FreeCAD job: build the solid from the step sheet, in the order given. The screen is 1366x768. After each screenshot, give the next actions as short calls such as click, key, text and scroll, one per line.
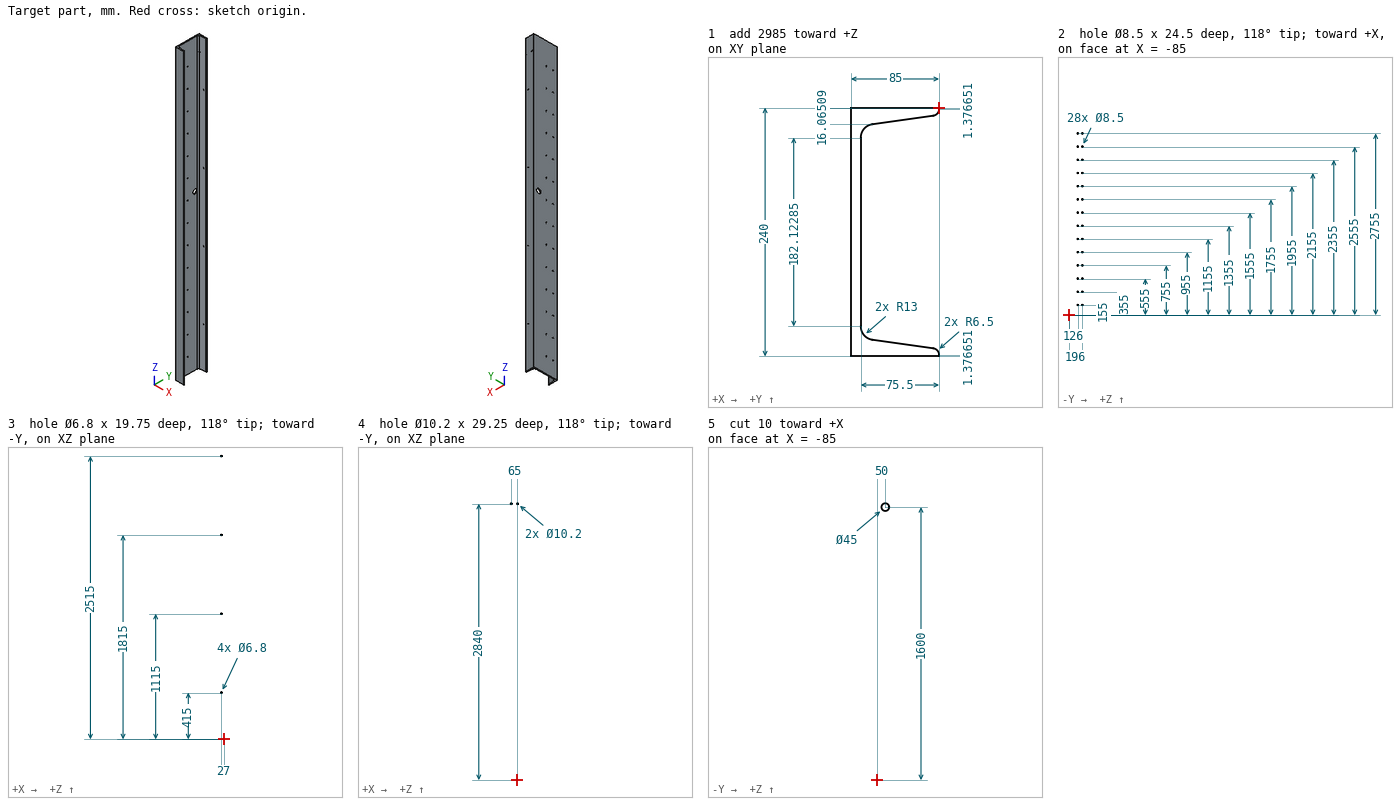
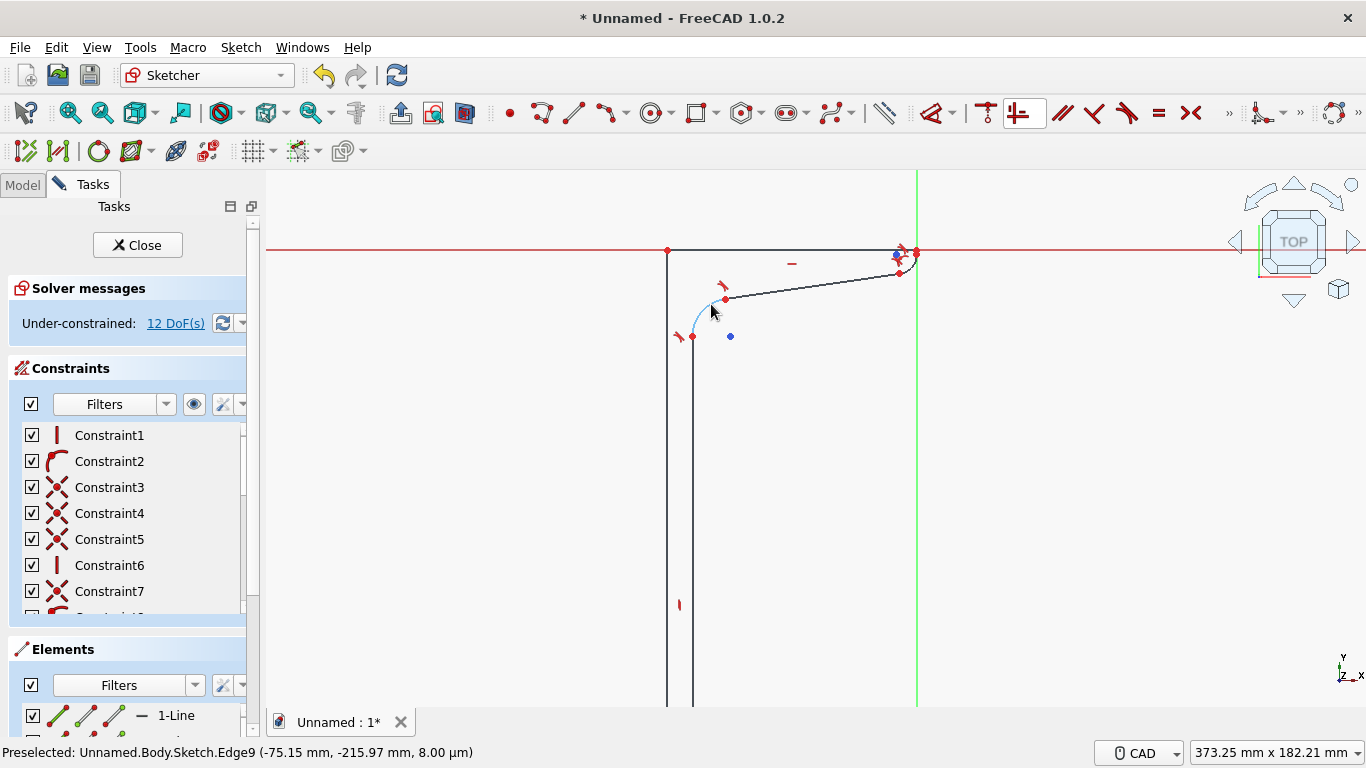
click(710, 305)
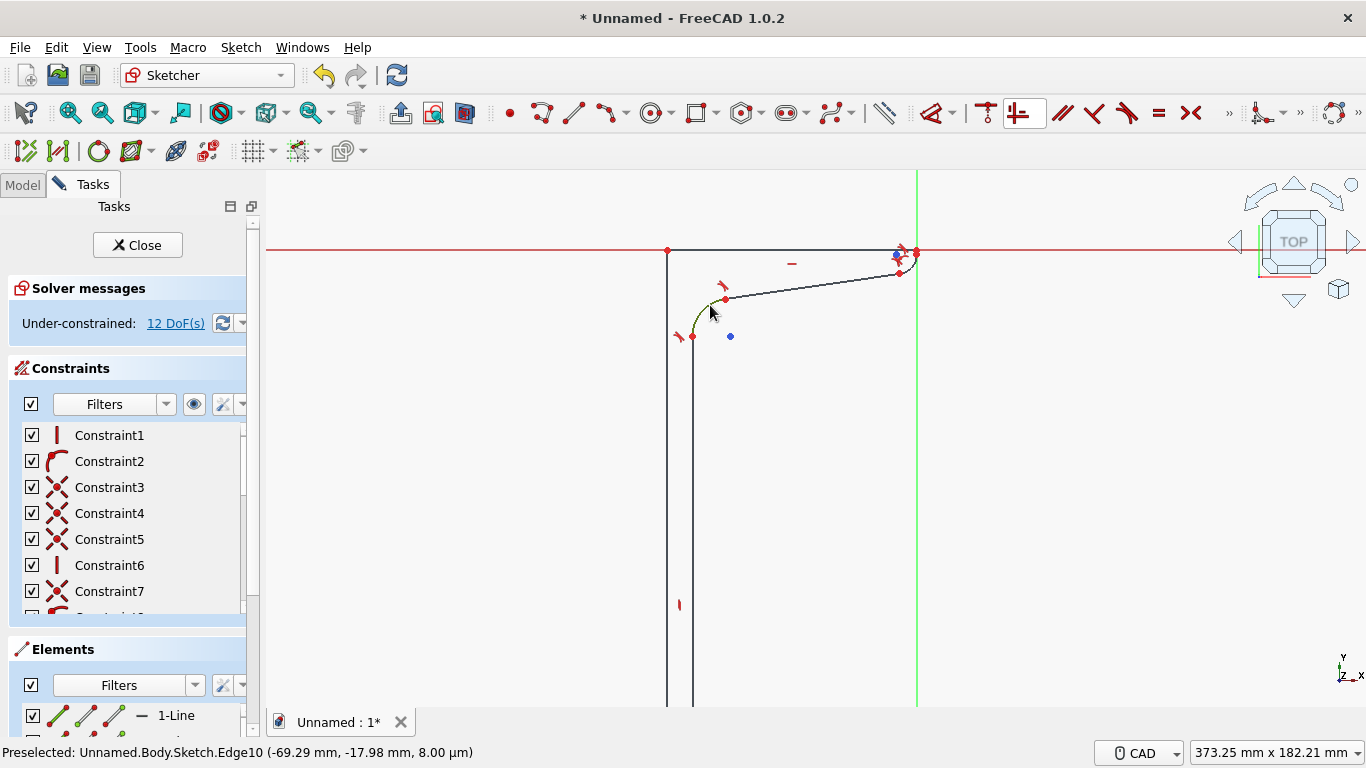
click(1160, 114)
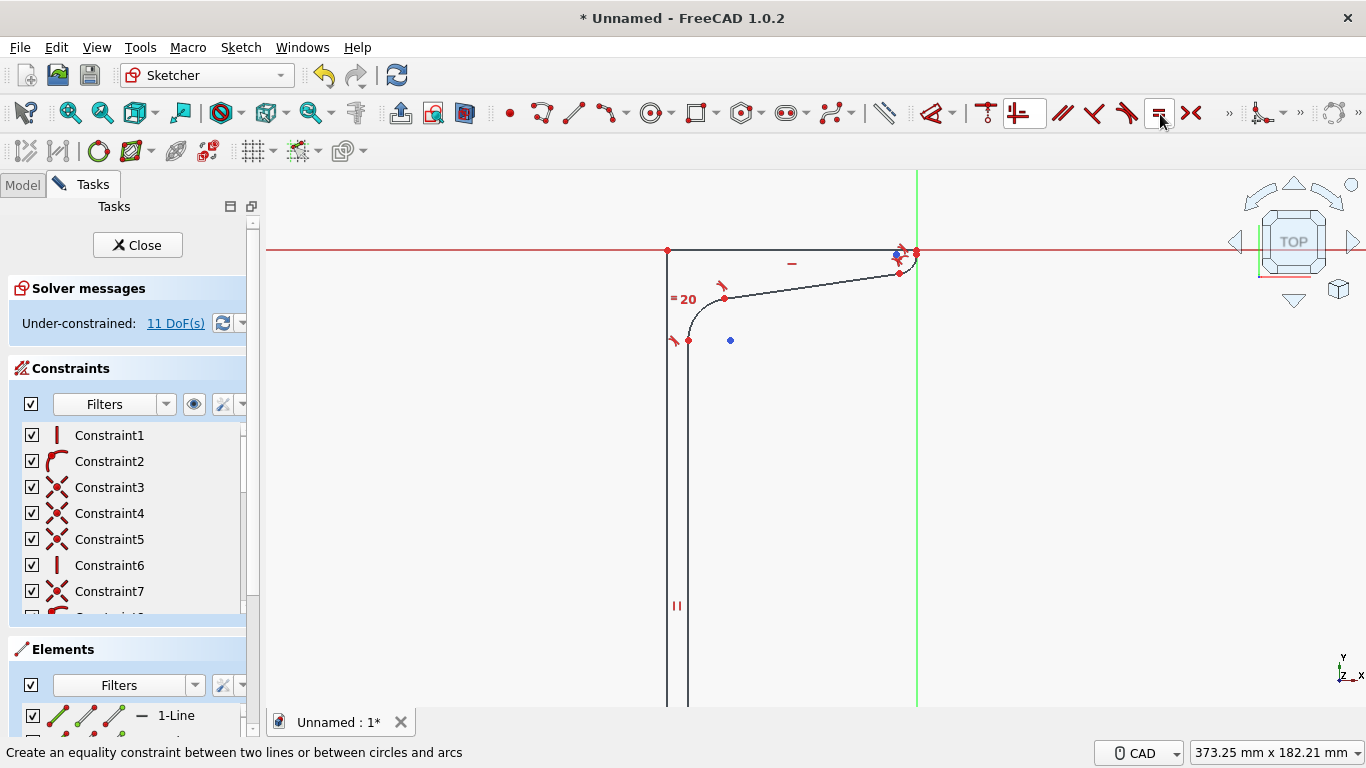
scroll(915, 262, up, 3)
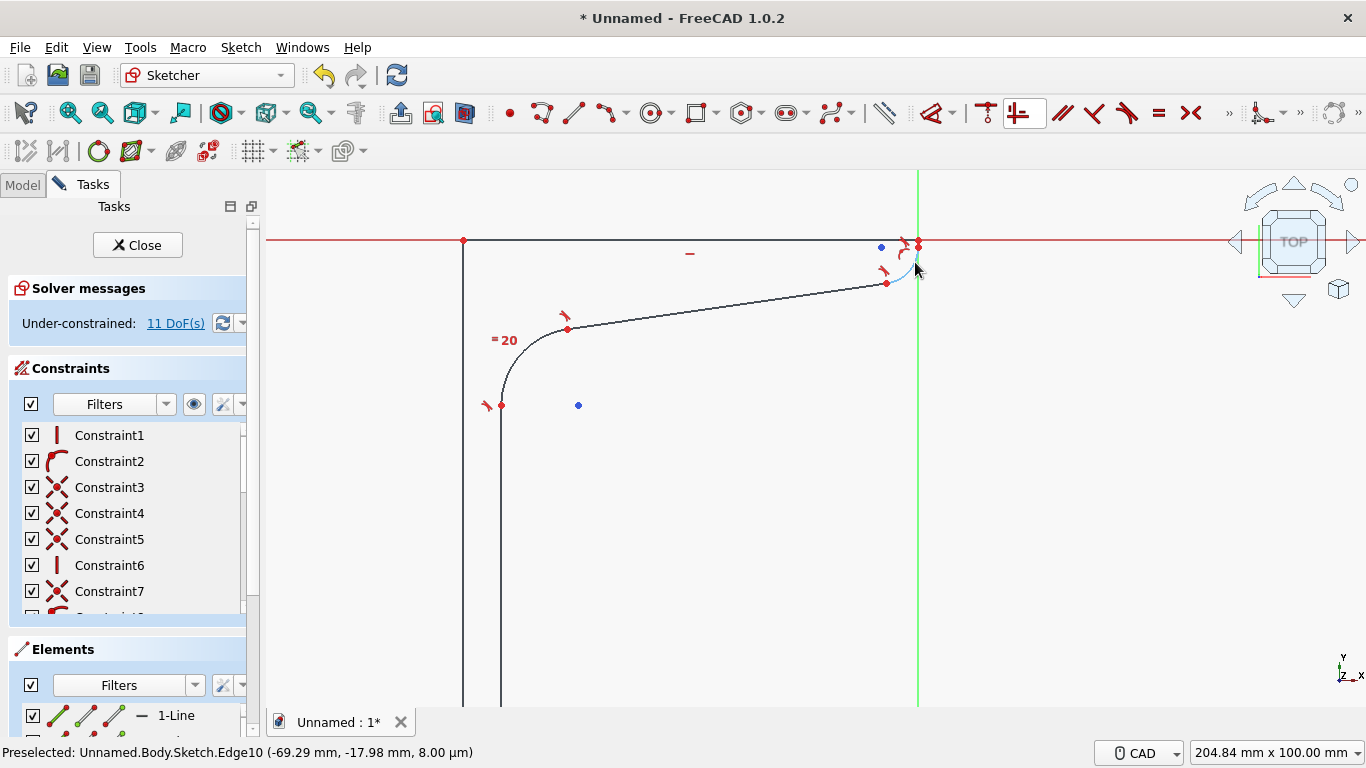
click(915, 263)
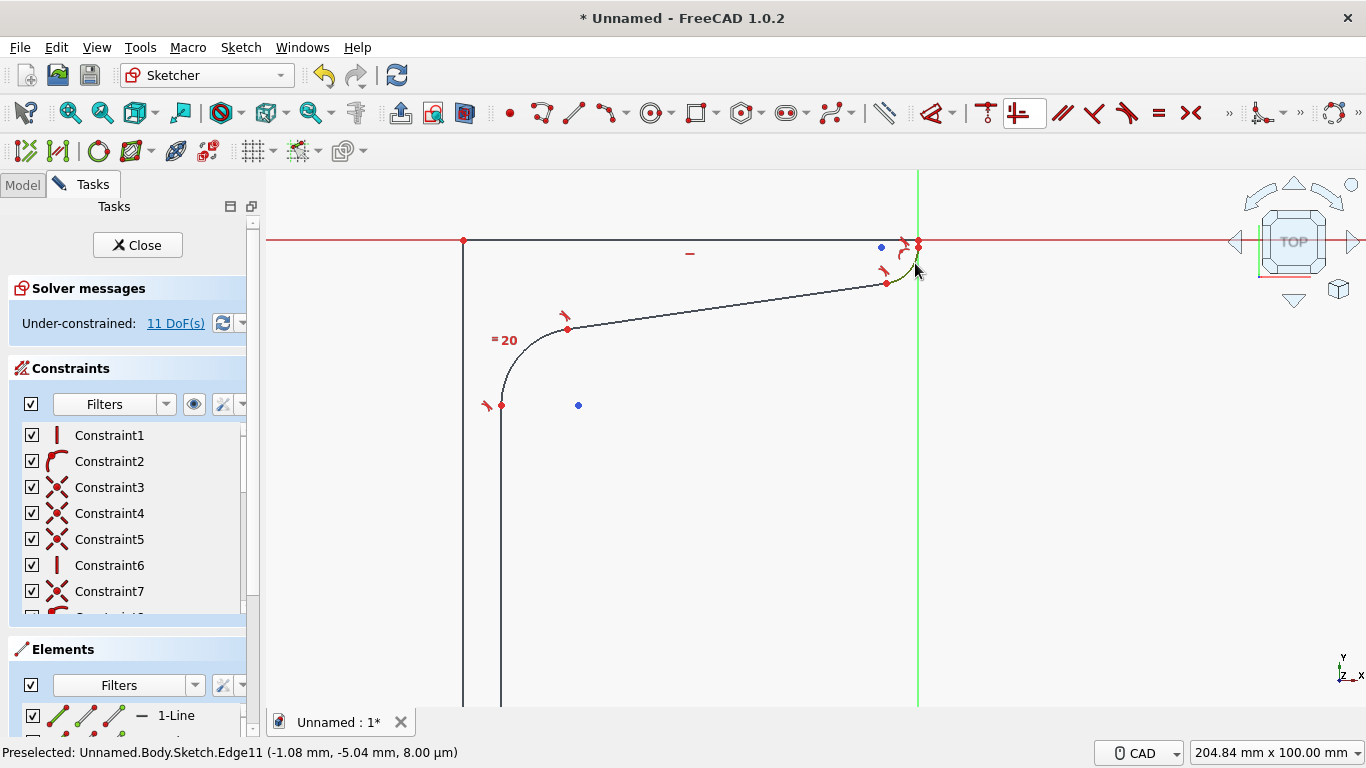
scroll(766, 293, down, 7)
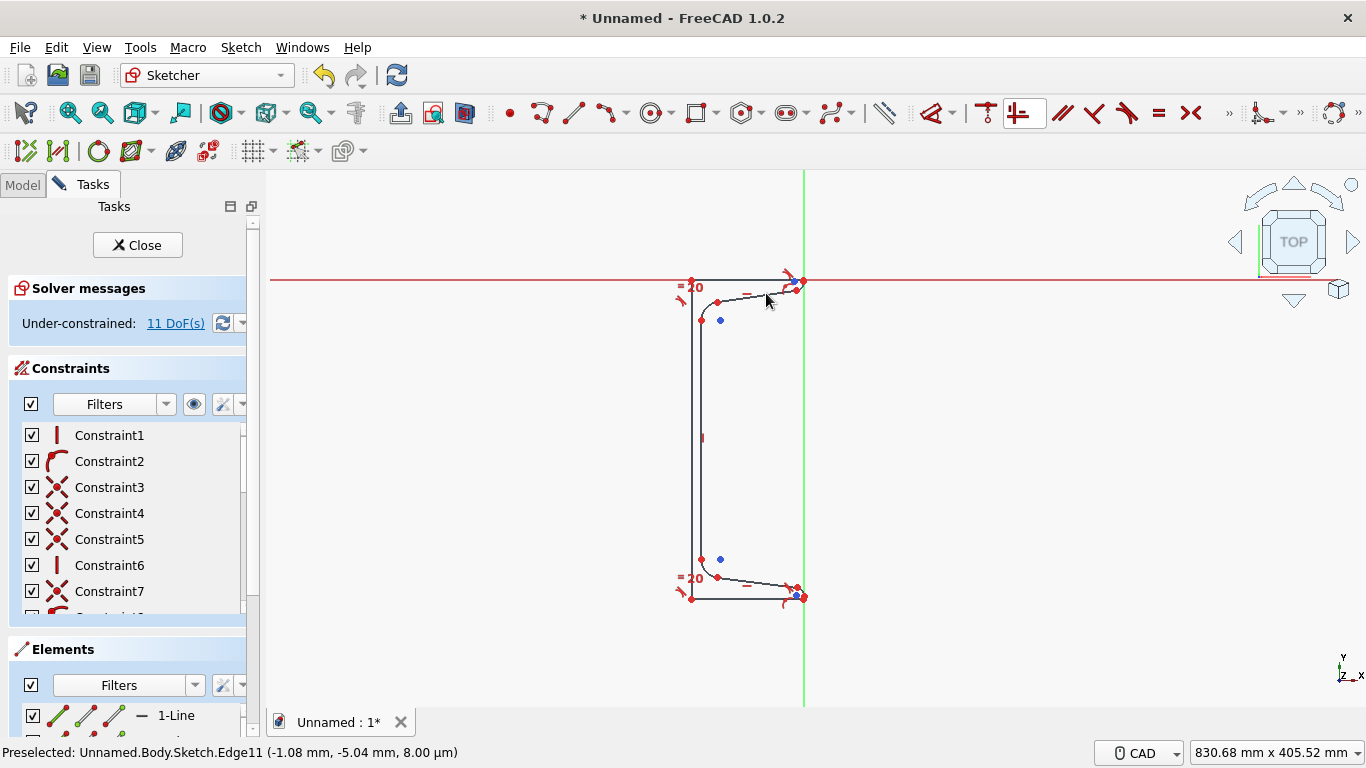
scroll(803, 593, up, 7)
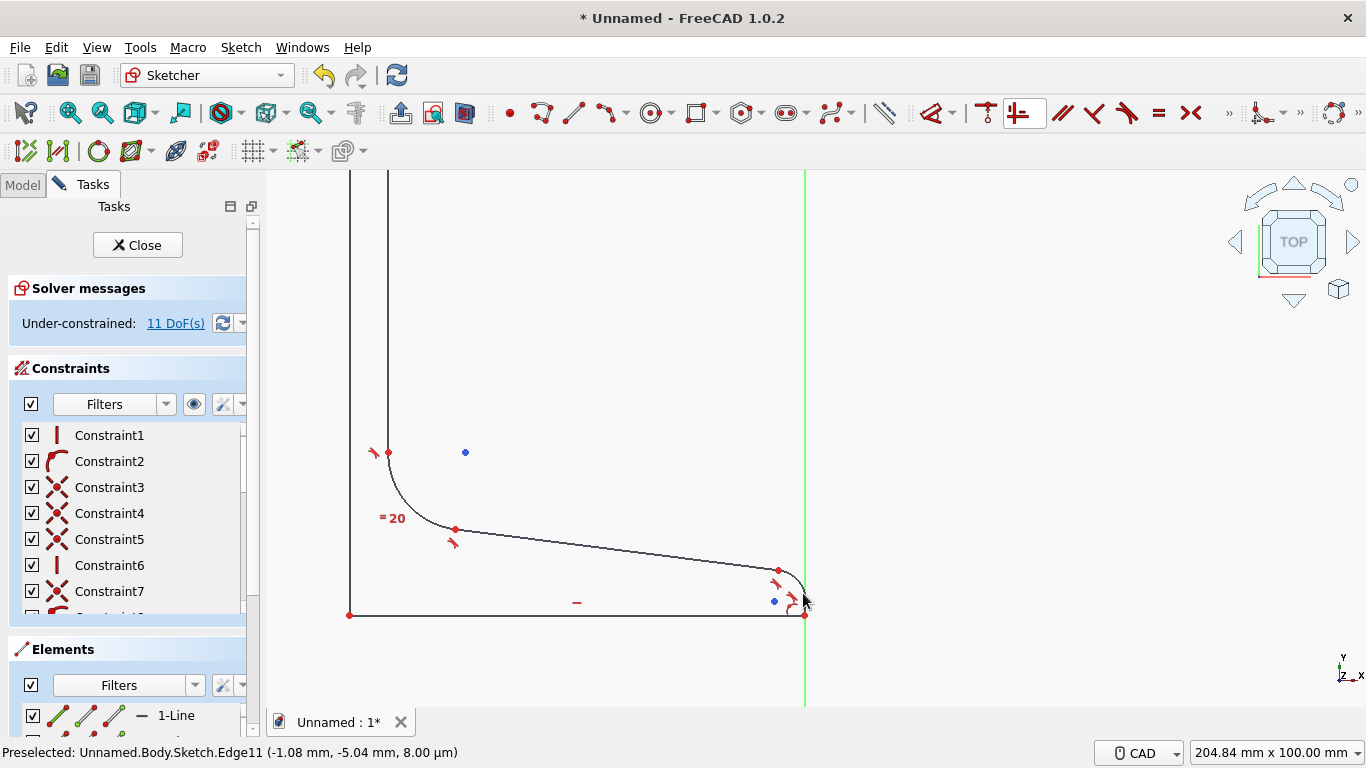
click(803, 589)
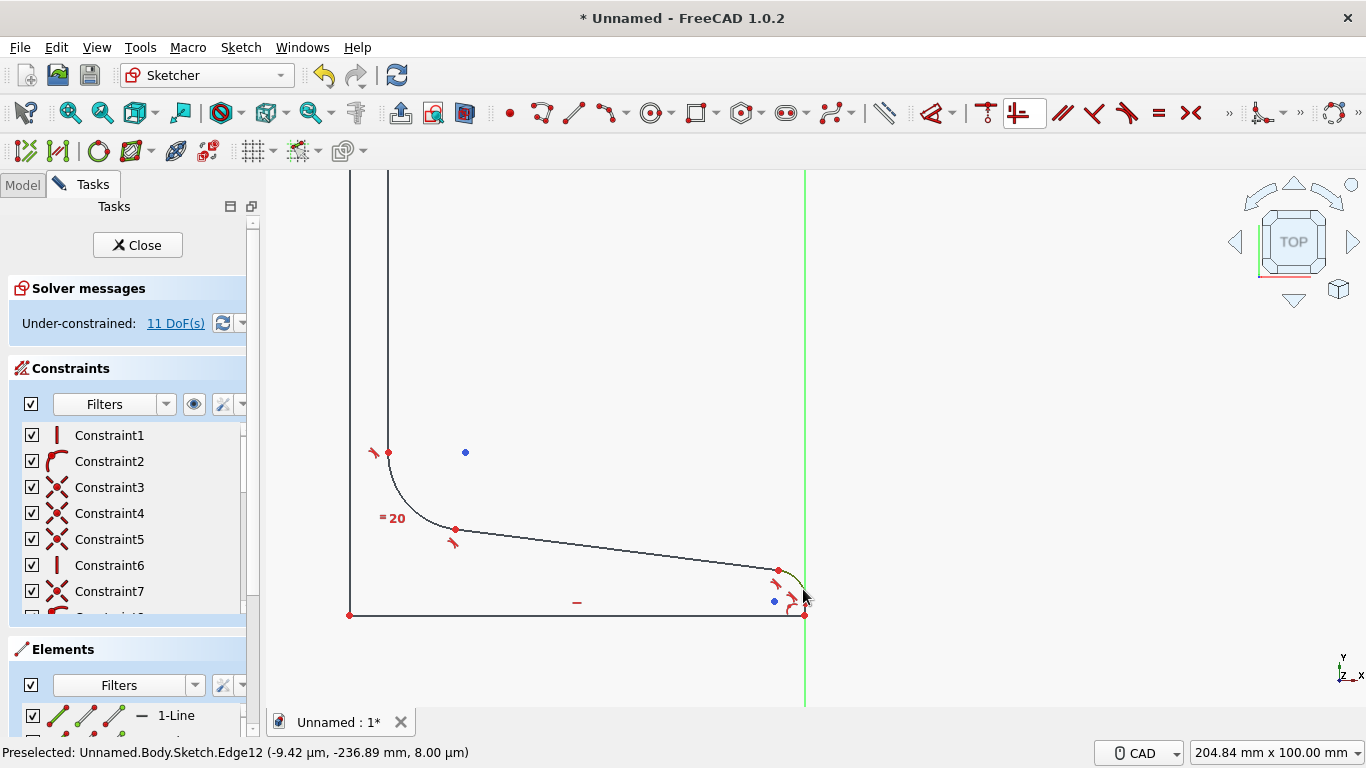
click(1160, 114)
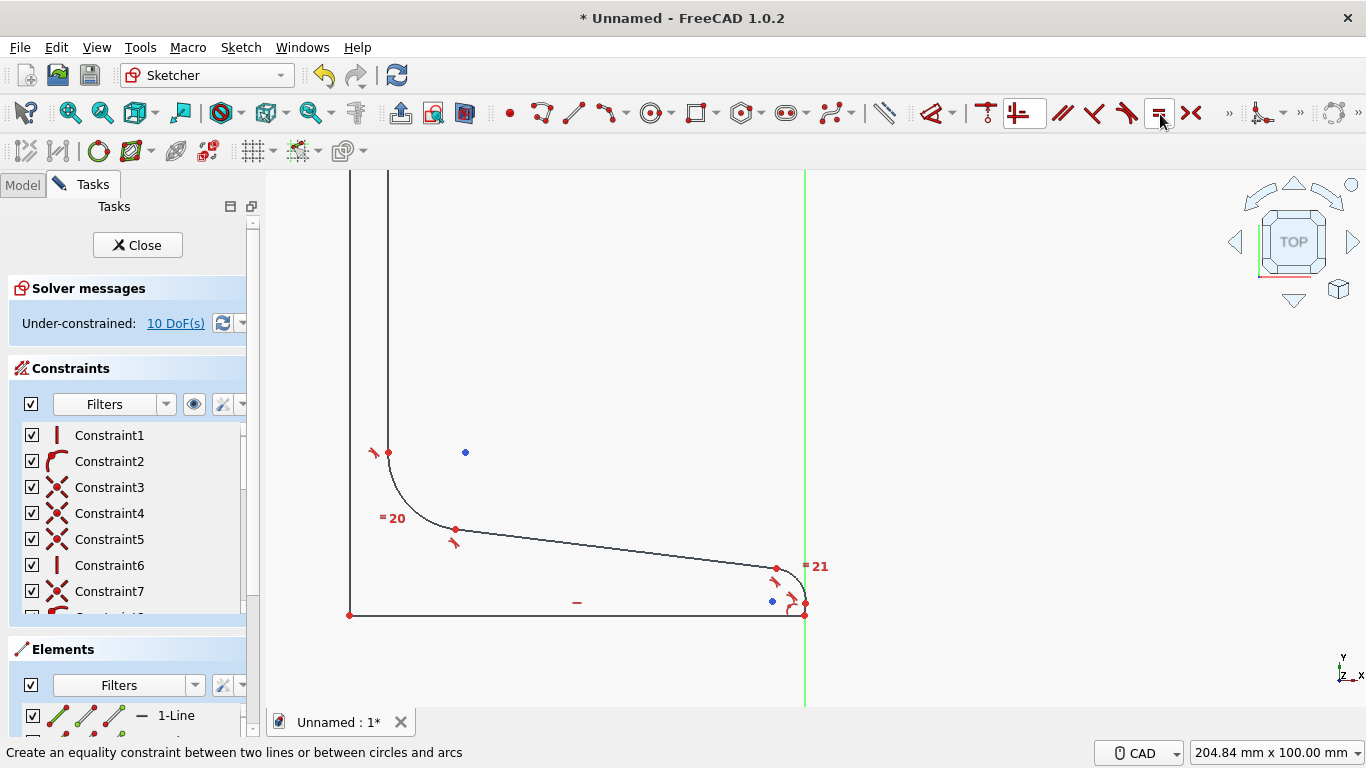
click(932, 114)